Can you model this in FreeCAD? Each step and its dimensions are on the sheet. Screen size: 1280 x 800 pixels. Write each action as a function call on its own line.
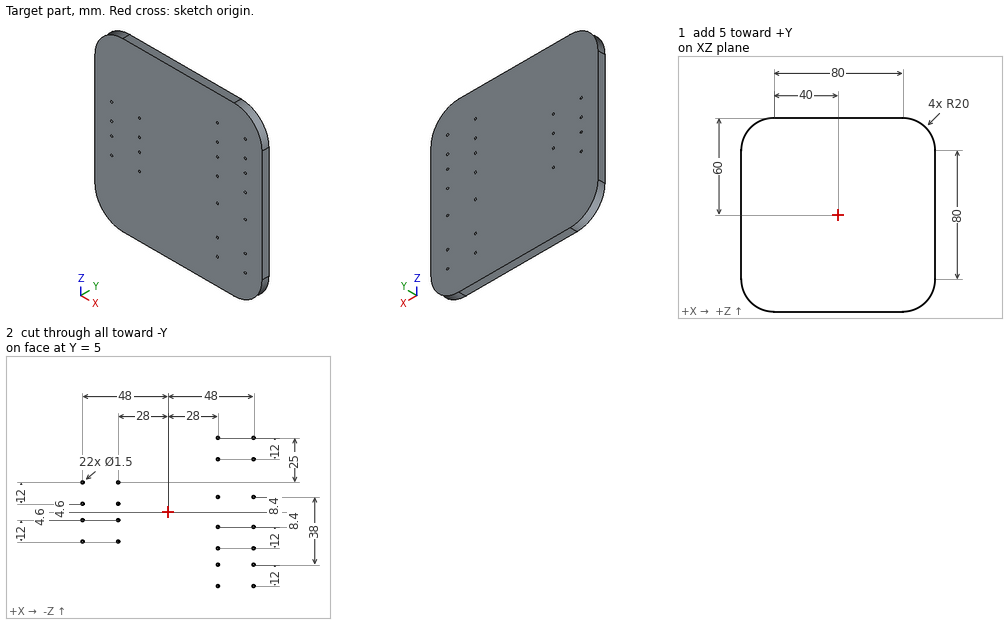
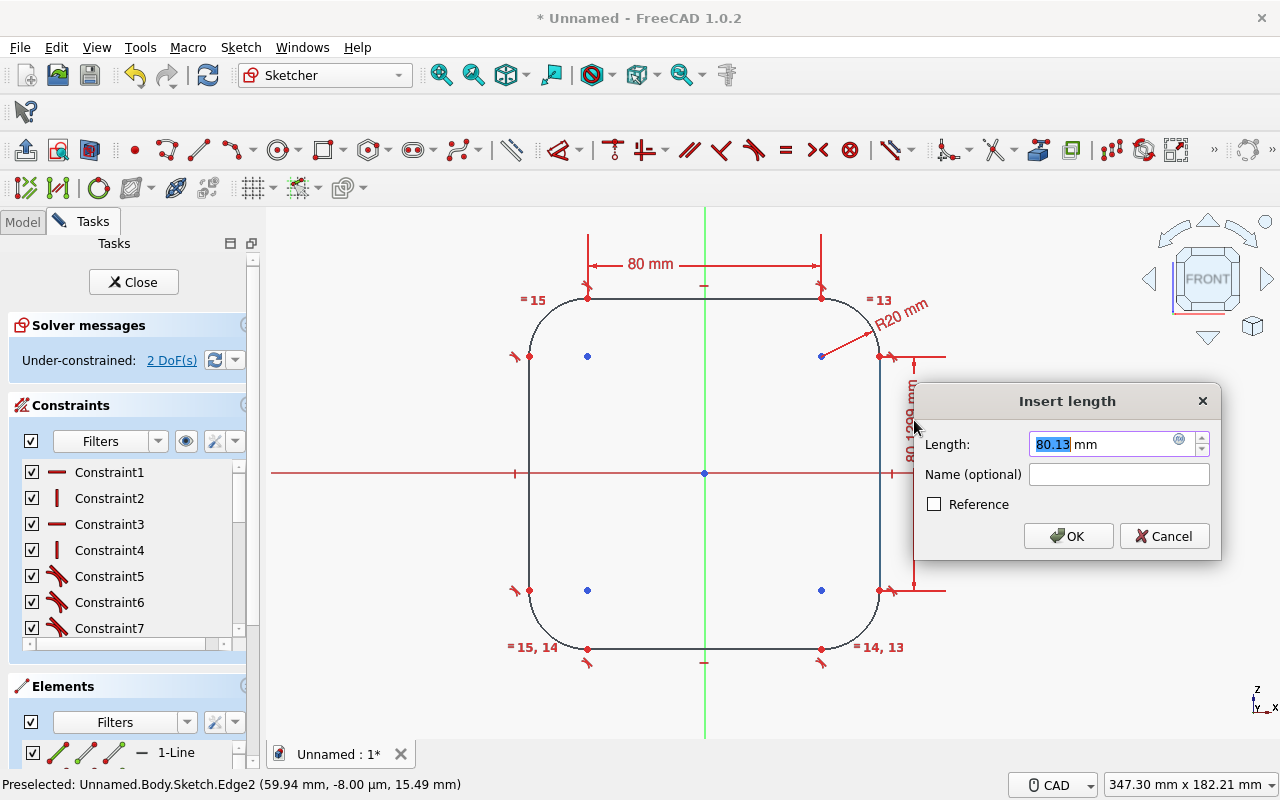
text(80)
key(Return)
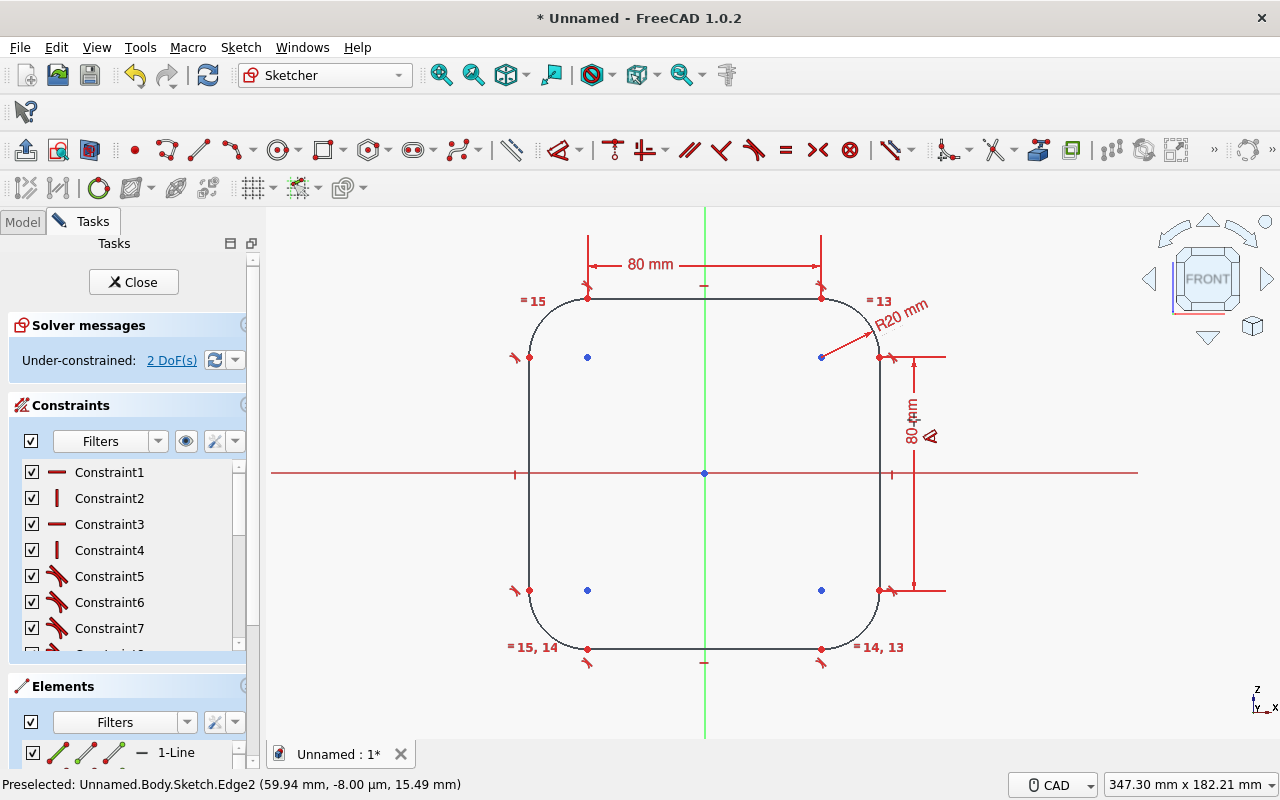
click(588, 299)
click(646, 507)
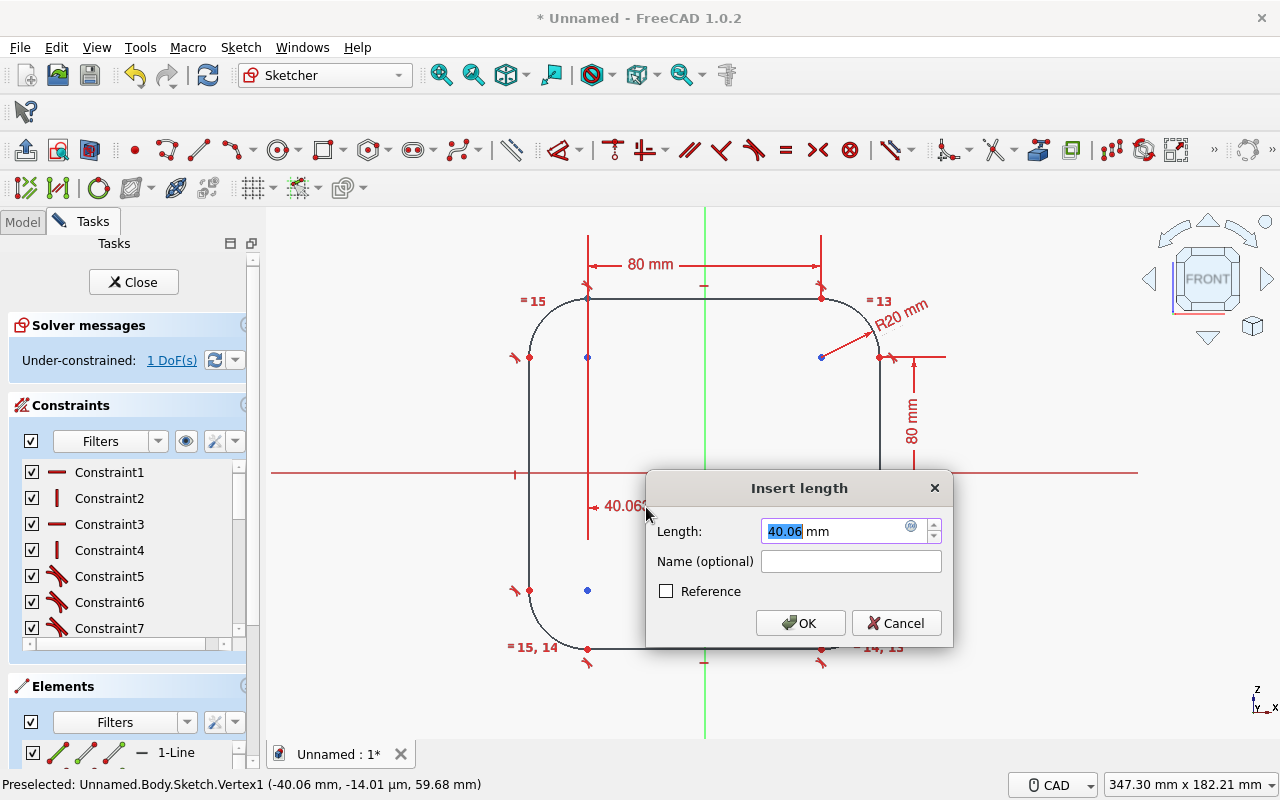
text(40)
key(Return)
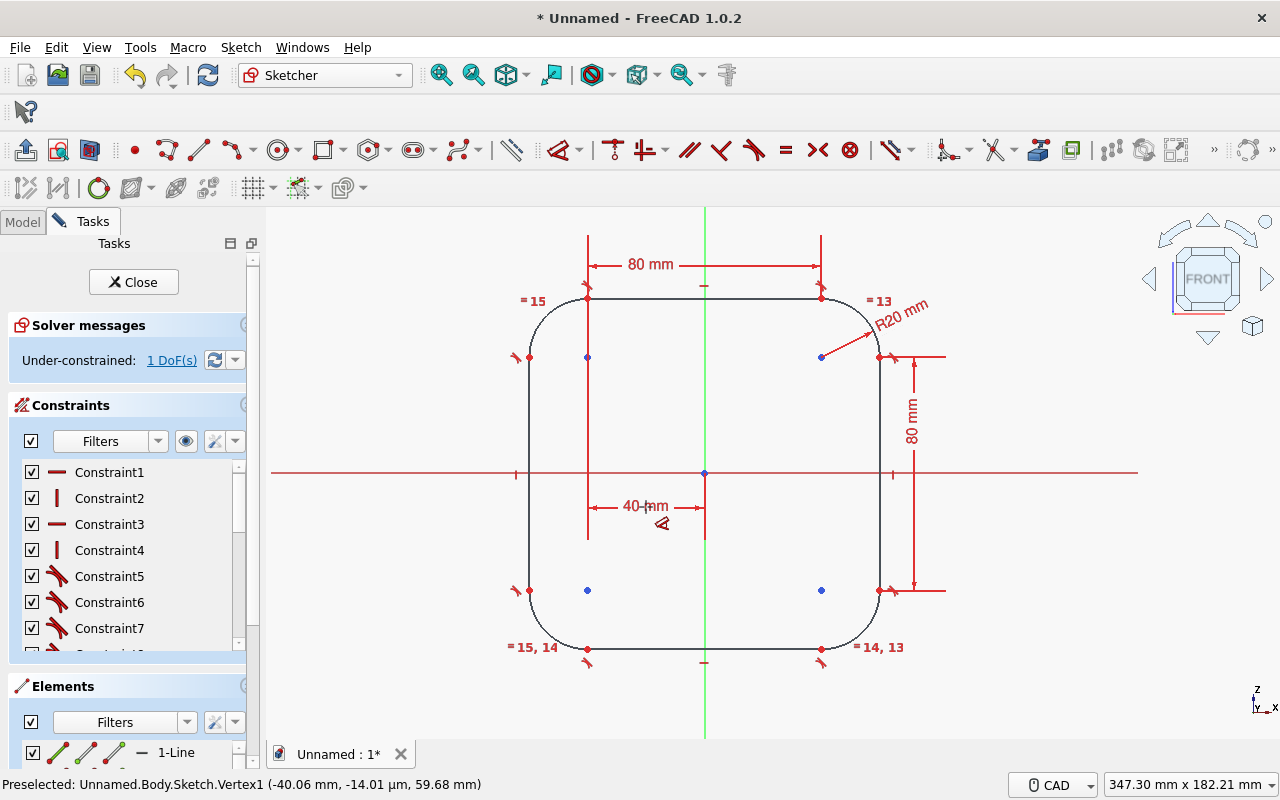
click(588, 299)
click(554, 386)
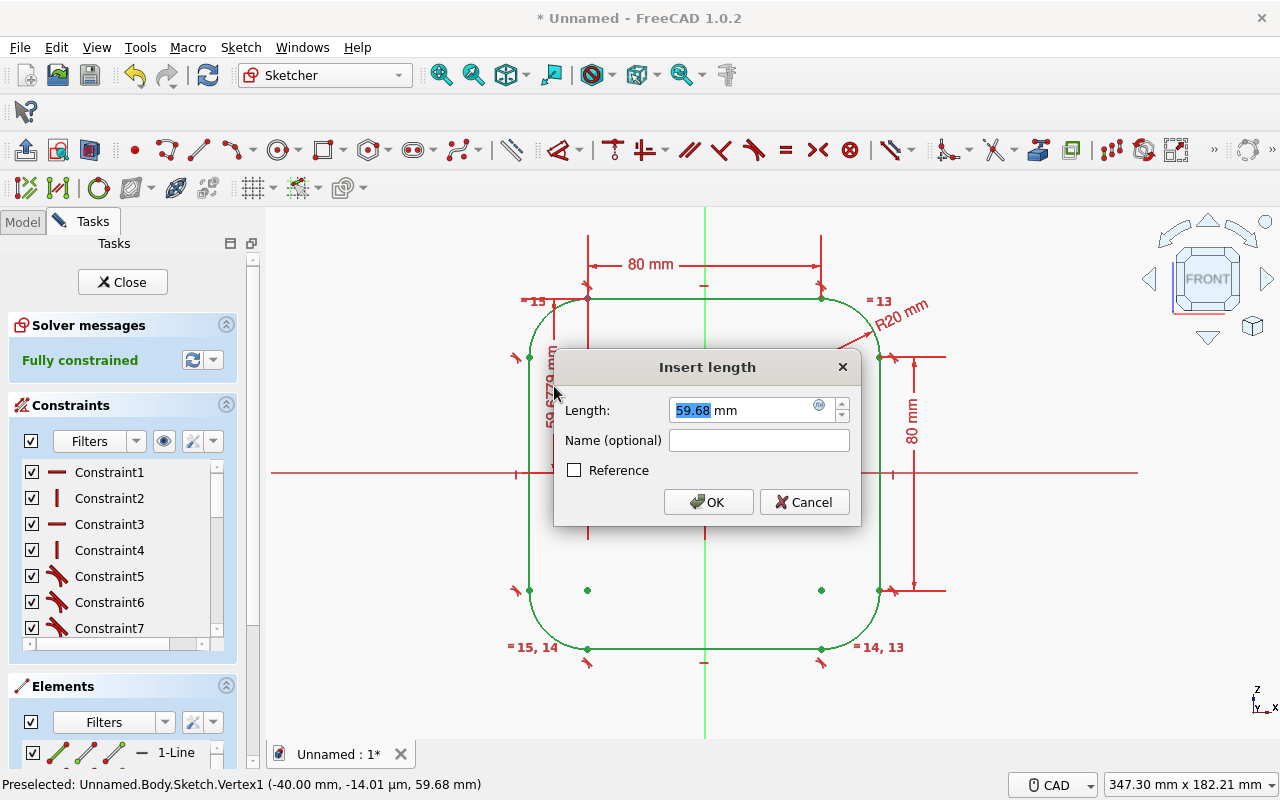
text(60)
key(Return)
key(Escape)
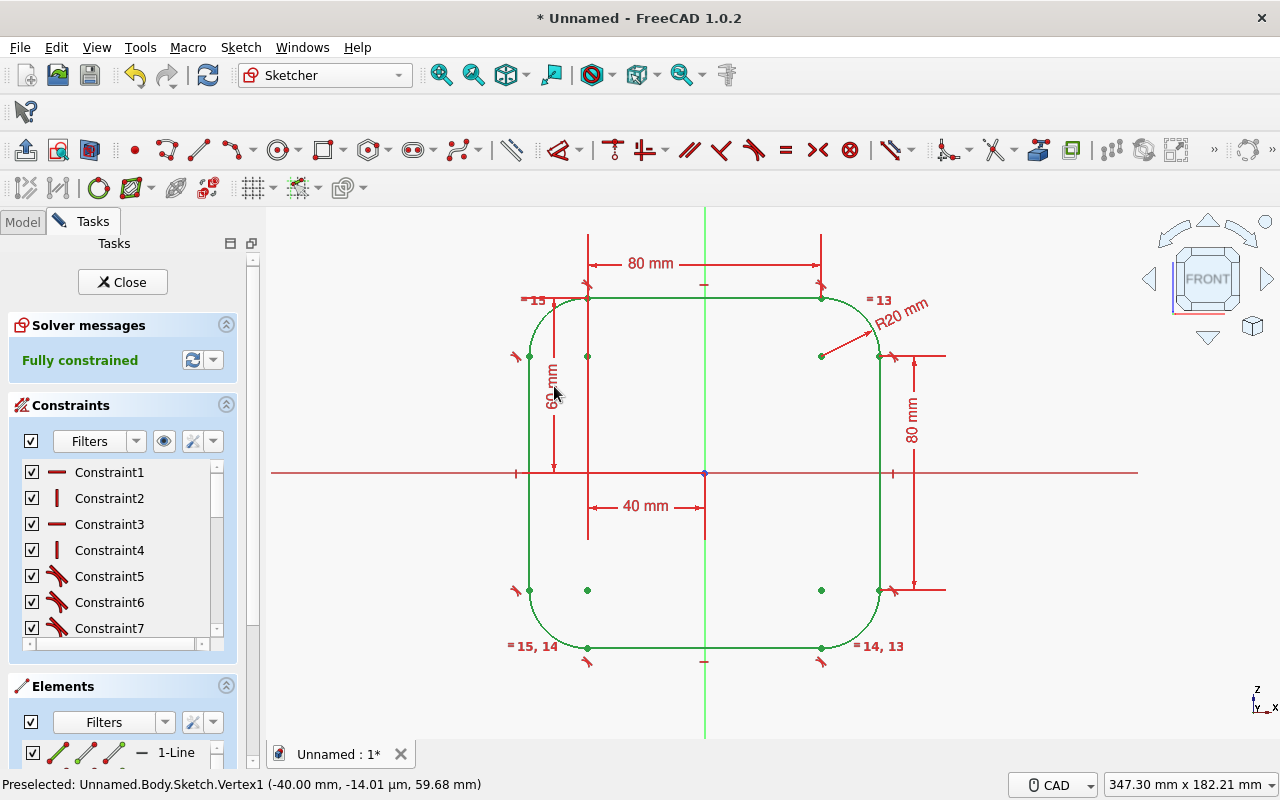
click(123, 282)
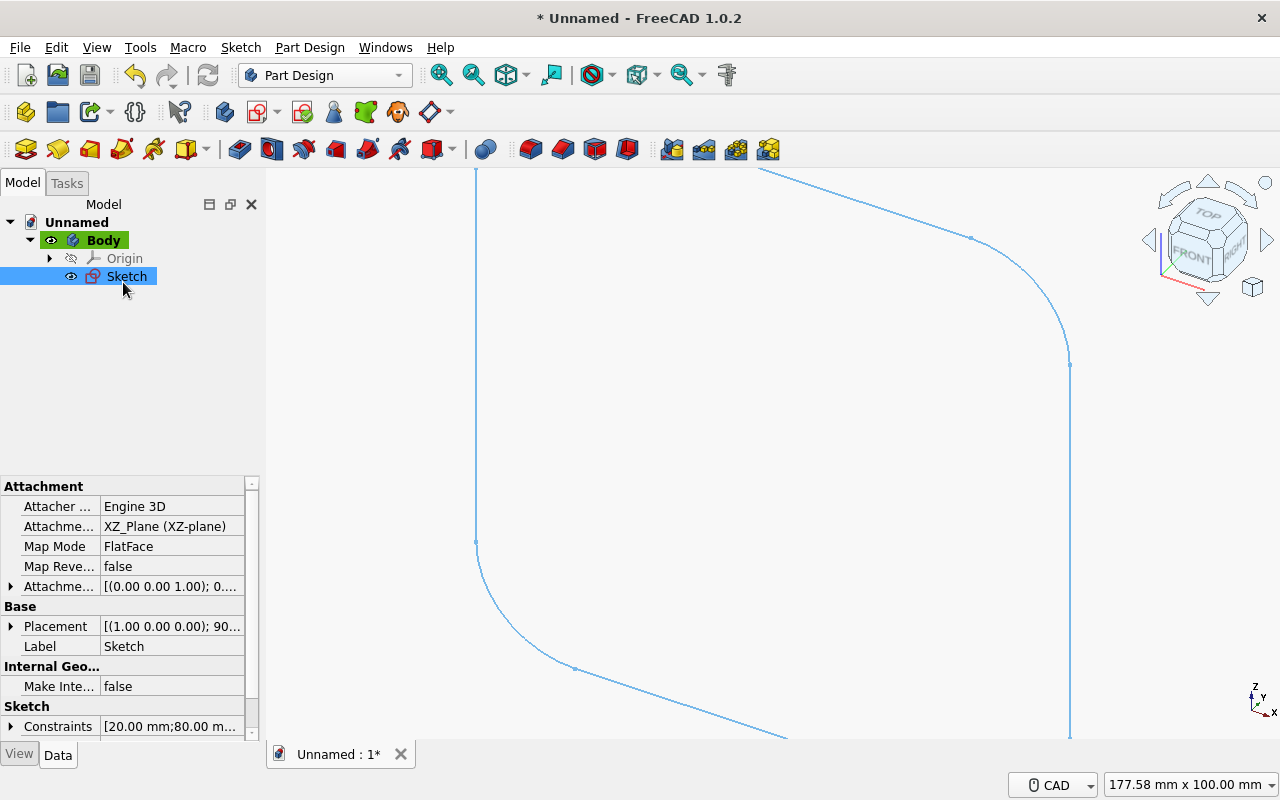
click(26, 150)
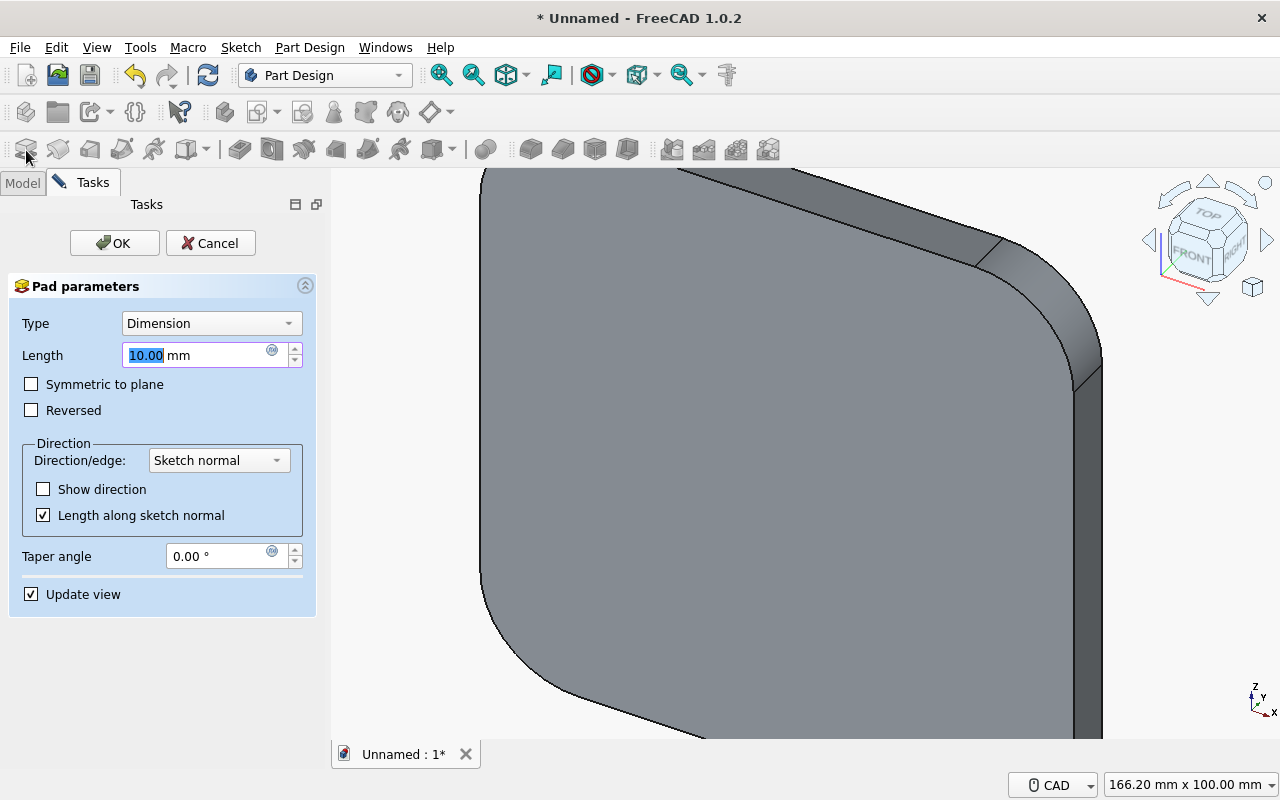
text(5)
key(Tab)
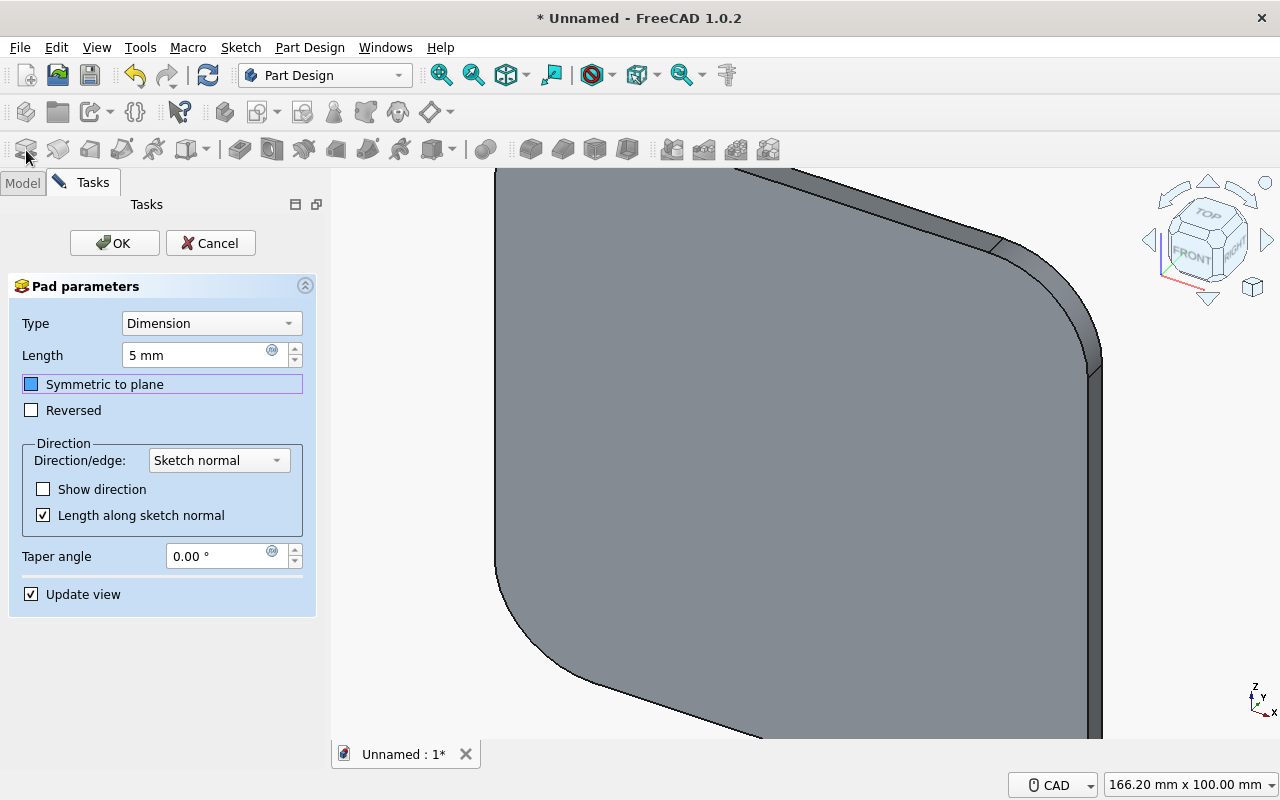
click(30, 410)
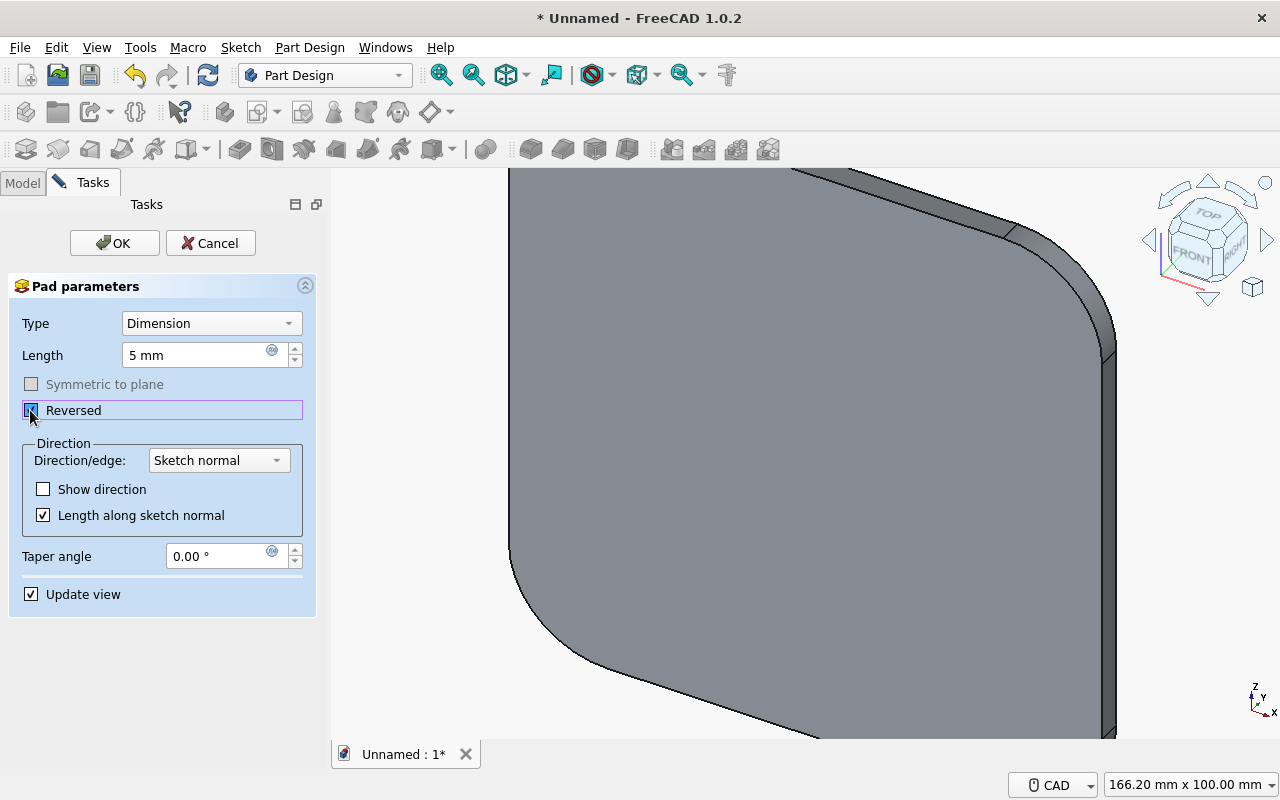
click(115, 243)